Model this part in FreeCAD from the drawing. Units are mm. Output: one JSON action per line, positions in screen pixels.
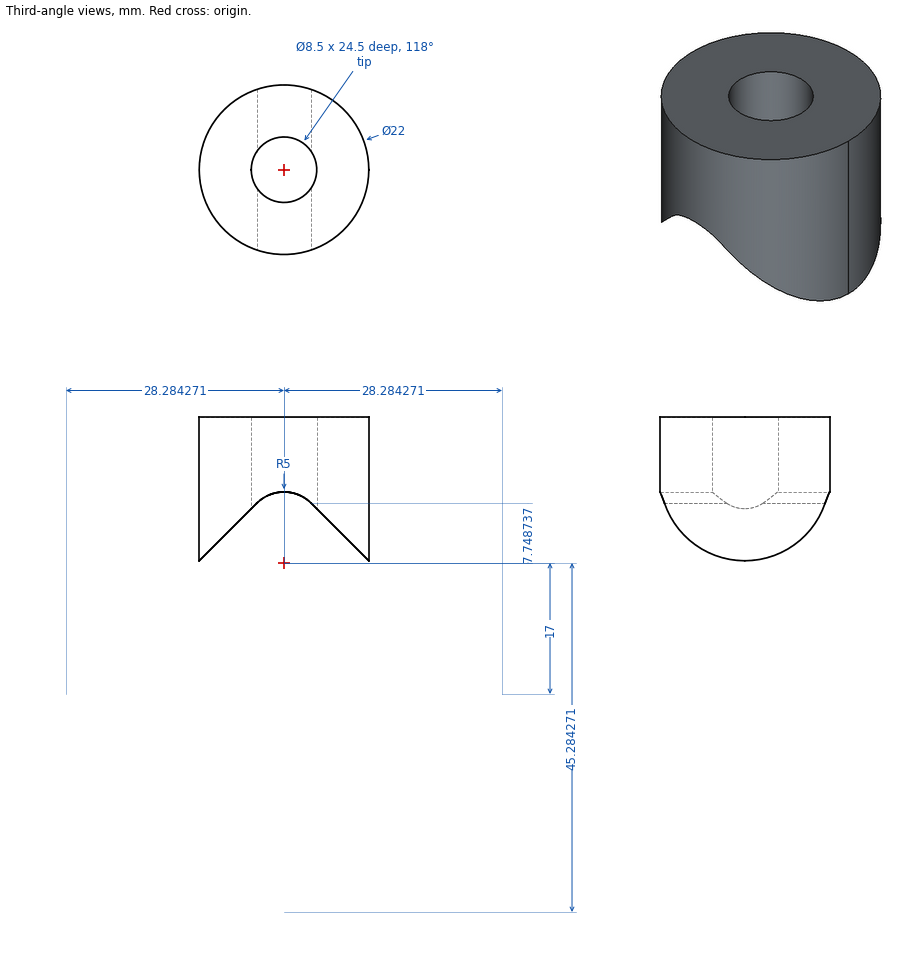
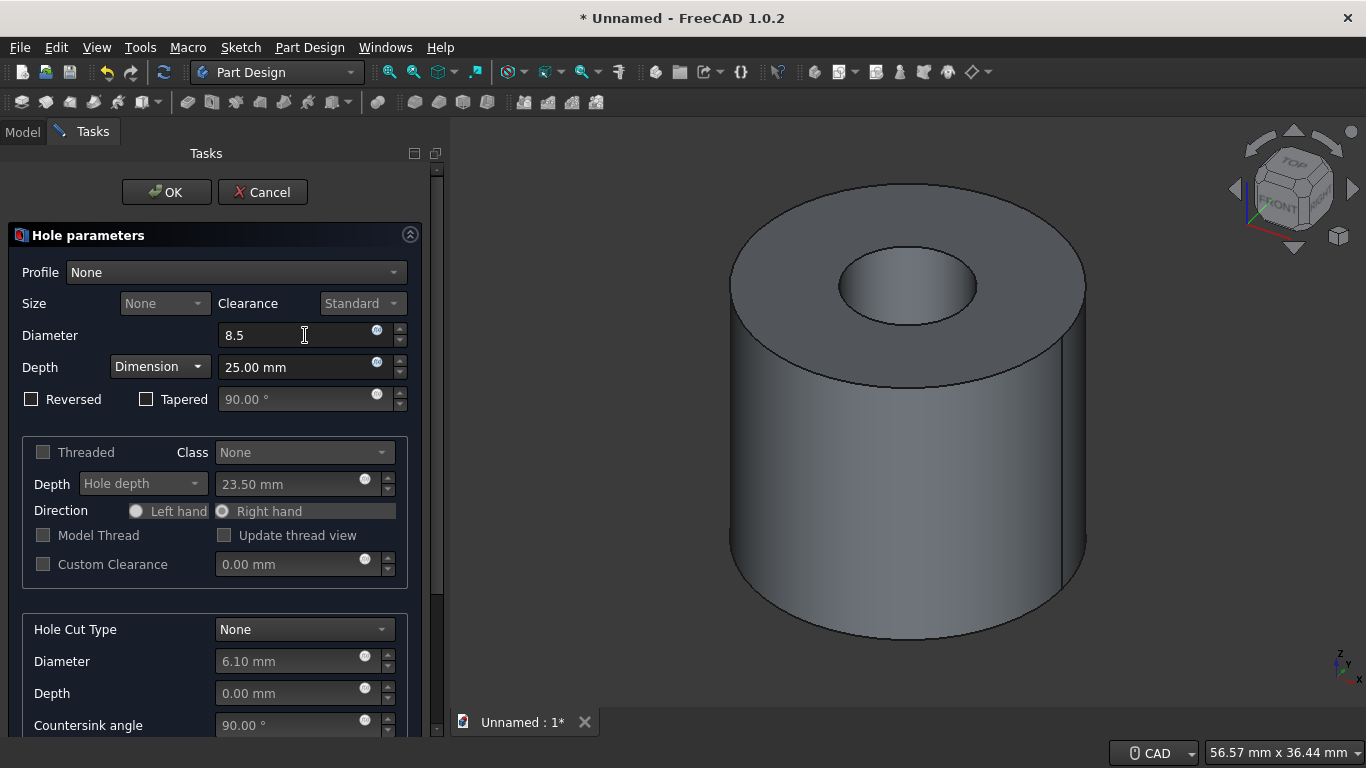
{"action": "triple_click", "coordinate": [305, 367]}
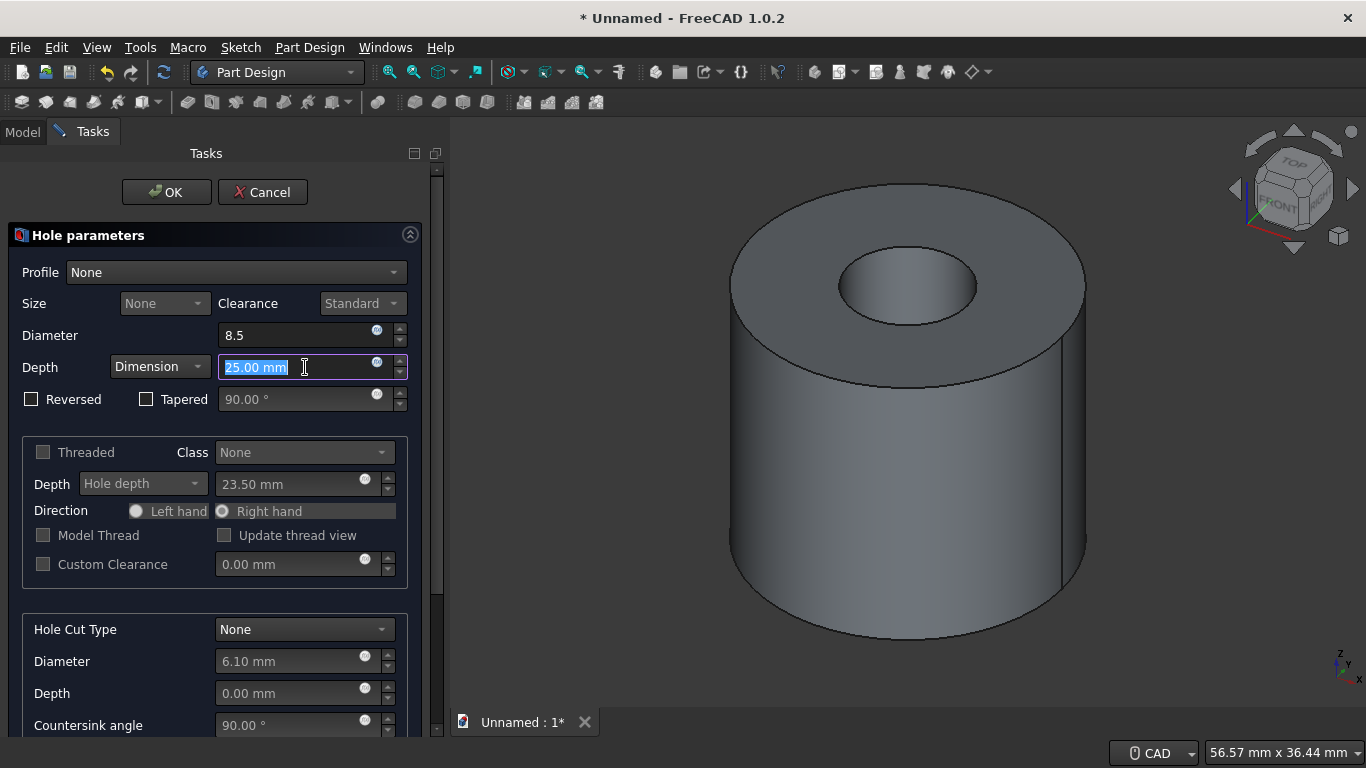
{"action": "type", "text": "24.5"}
{"action": "key", "text": "Tab"}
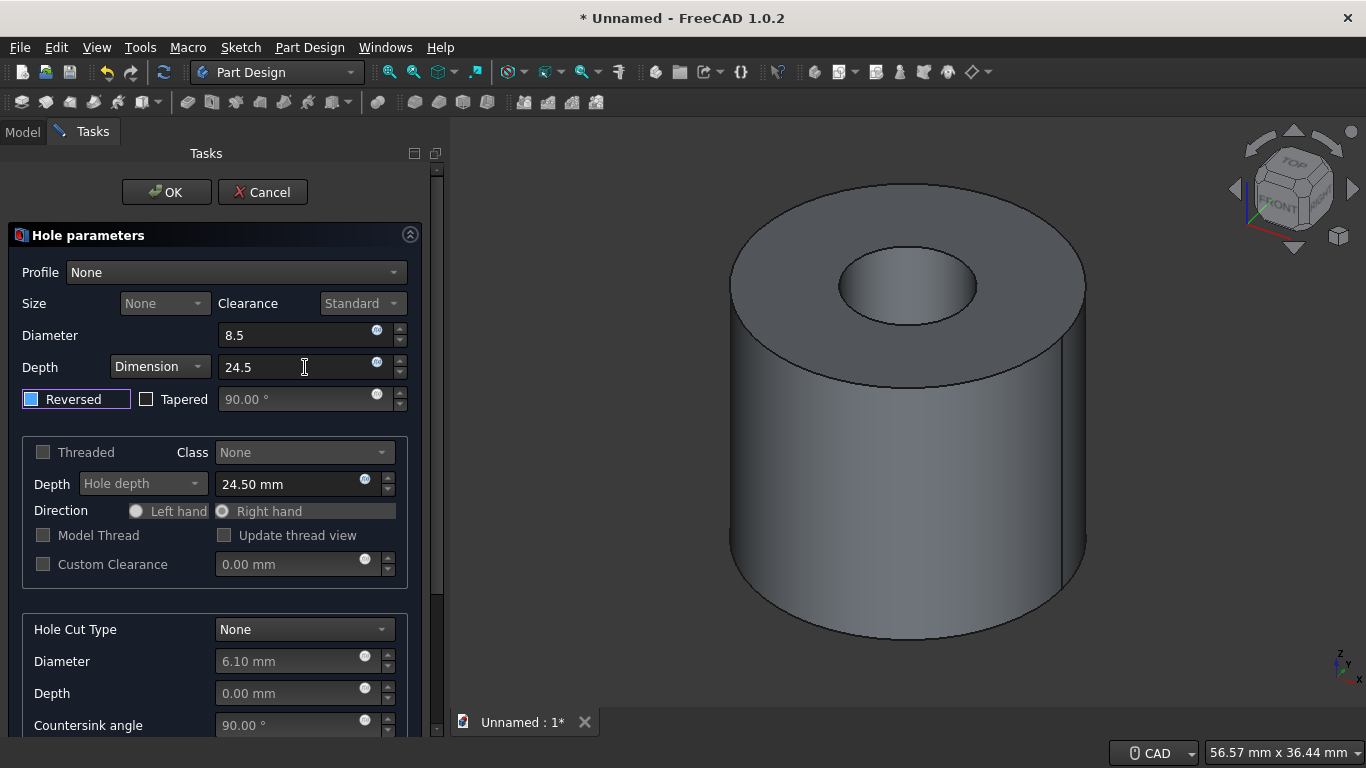
{"action": "left_click", "coordinate": [167, 192]}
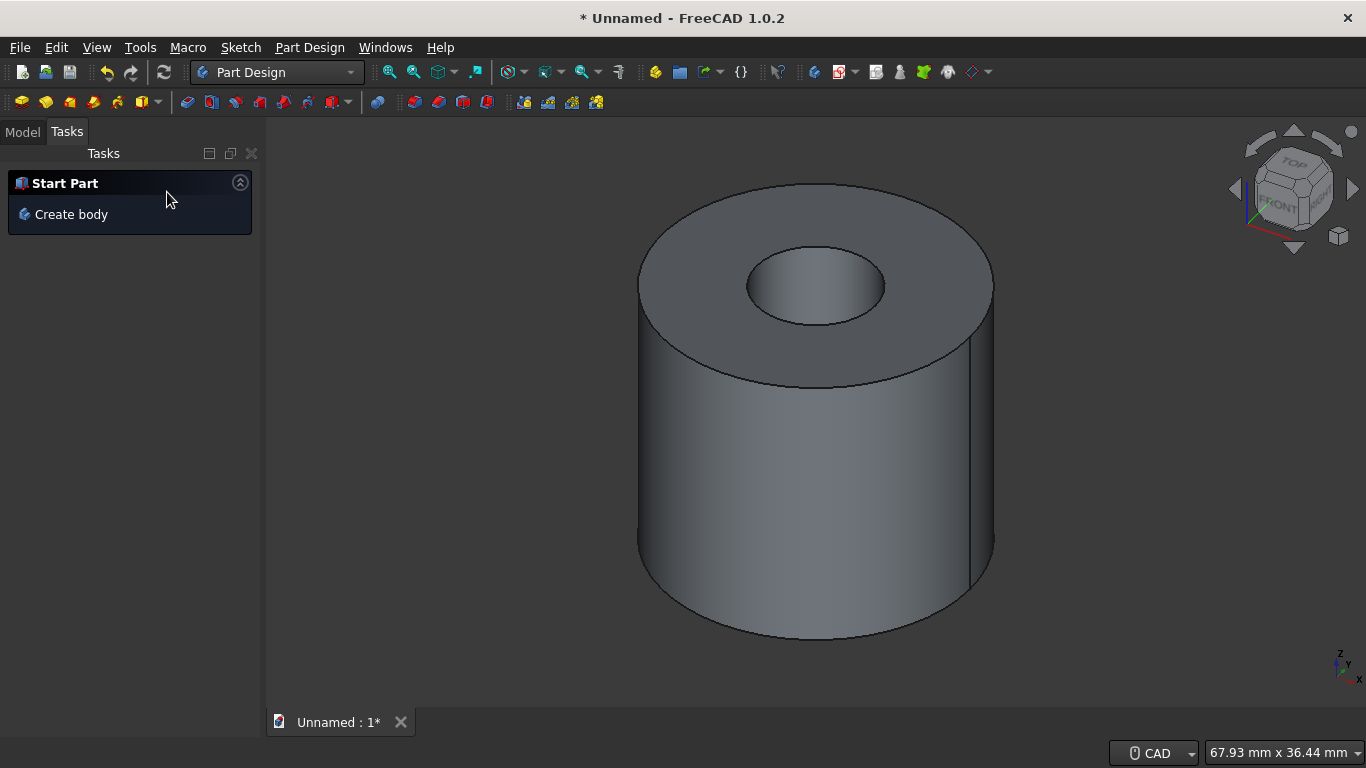
{"action": "left_click", "coordinate": [840, 72]}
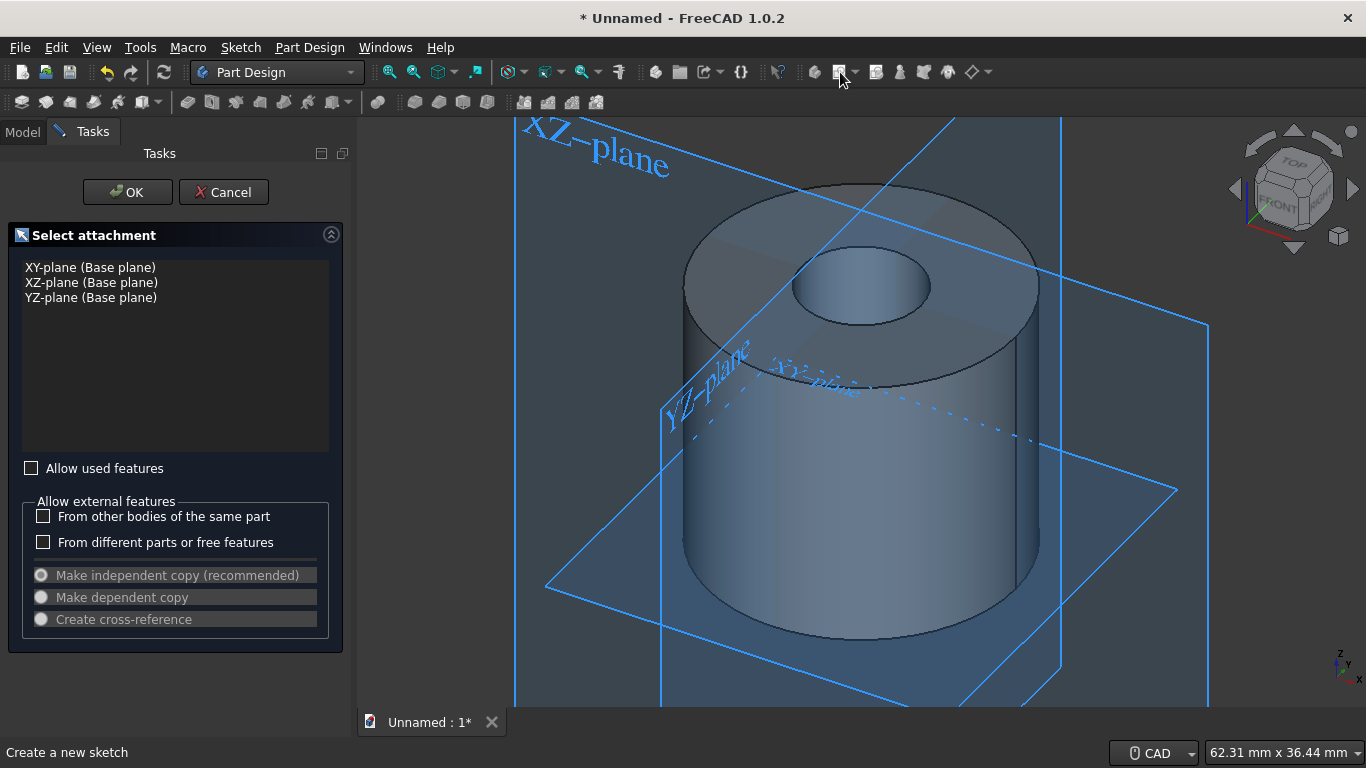
{"action": "left_click", "coordinate": [82, 282]}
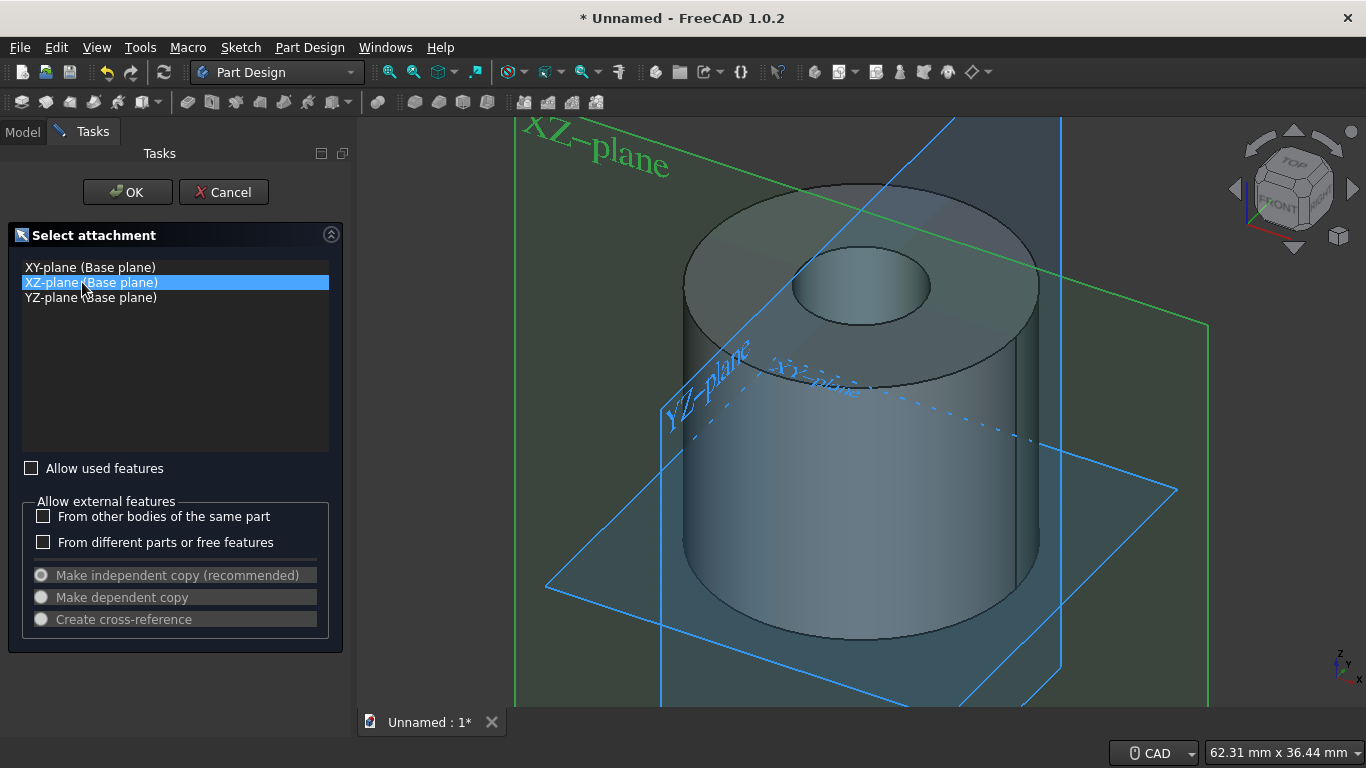
{"action": "left_click", "coordinate": [128, 192]}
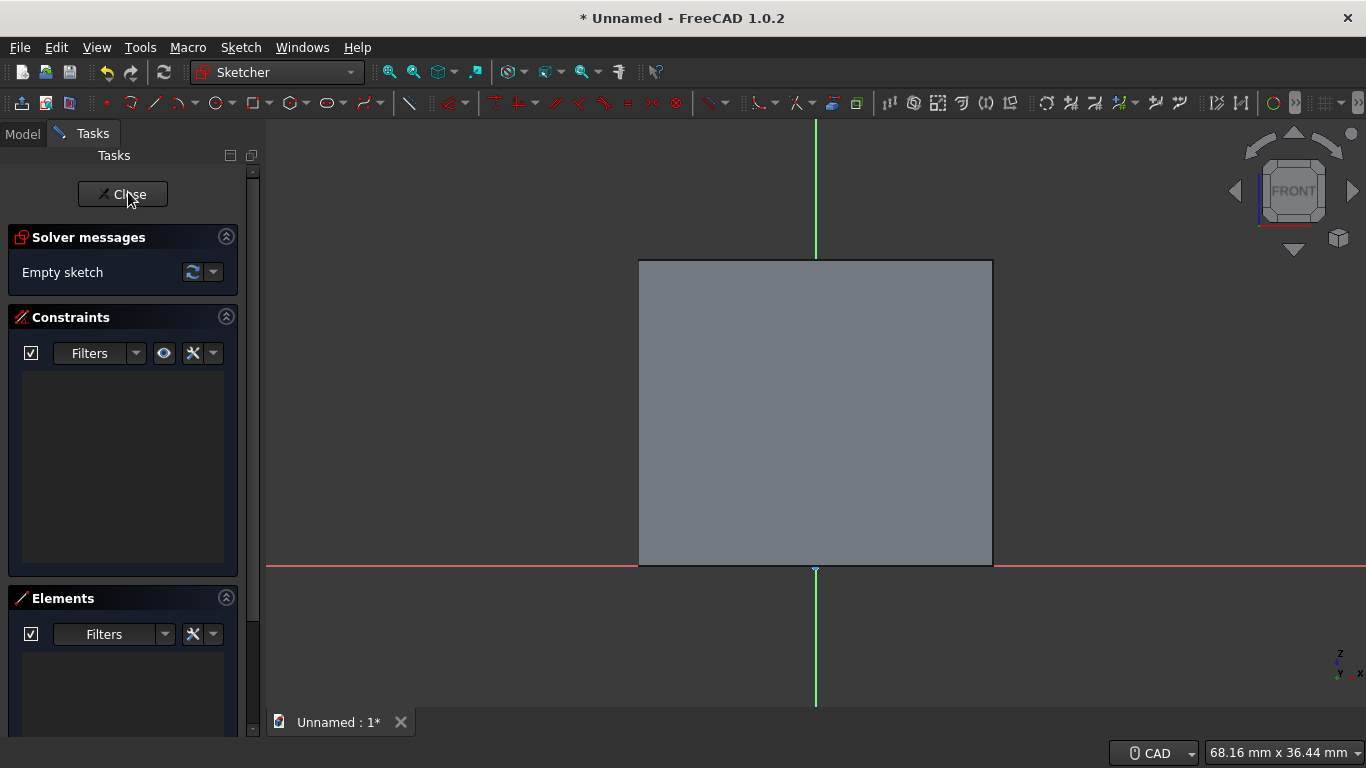
{"action": "key", "text": "q s"}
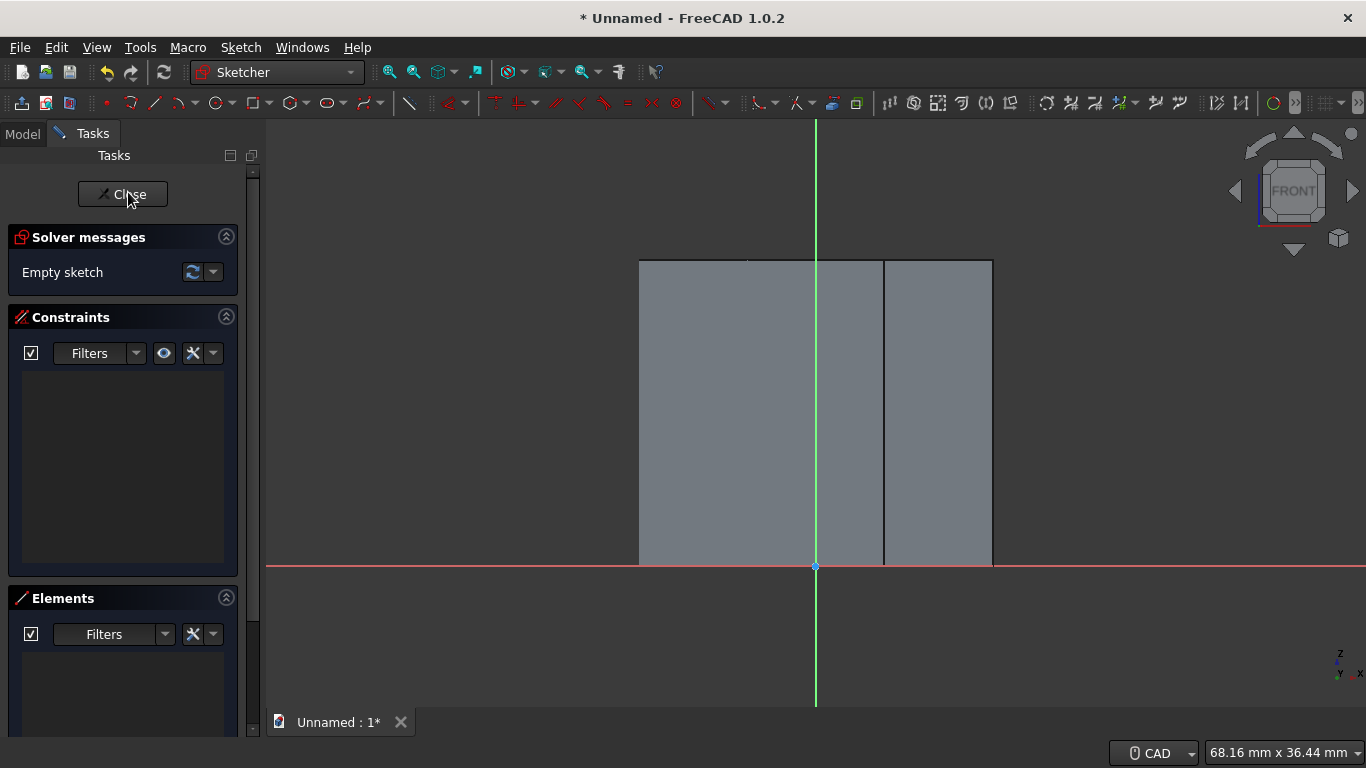
{"action": "scroll", "coordinate": [708, 154], "scroll_direction": "down", "scroll_amount": 5}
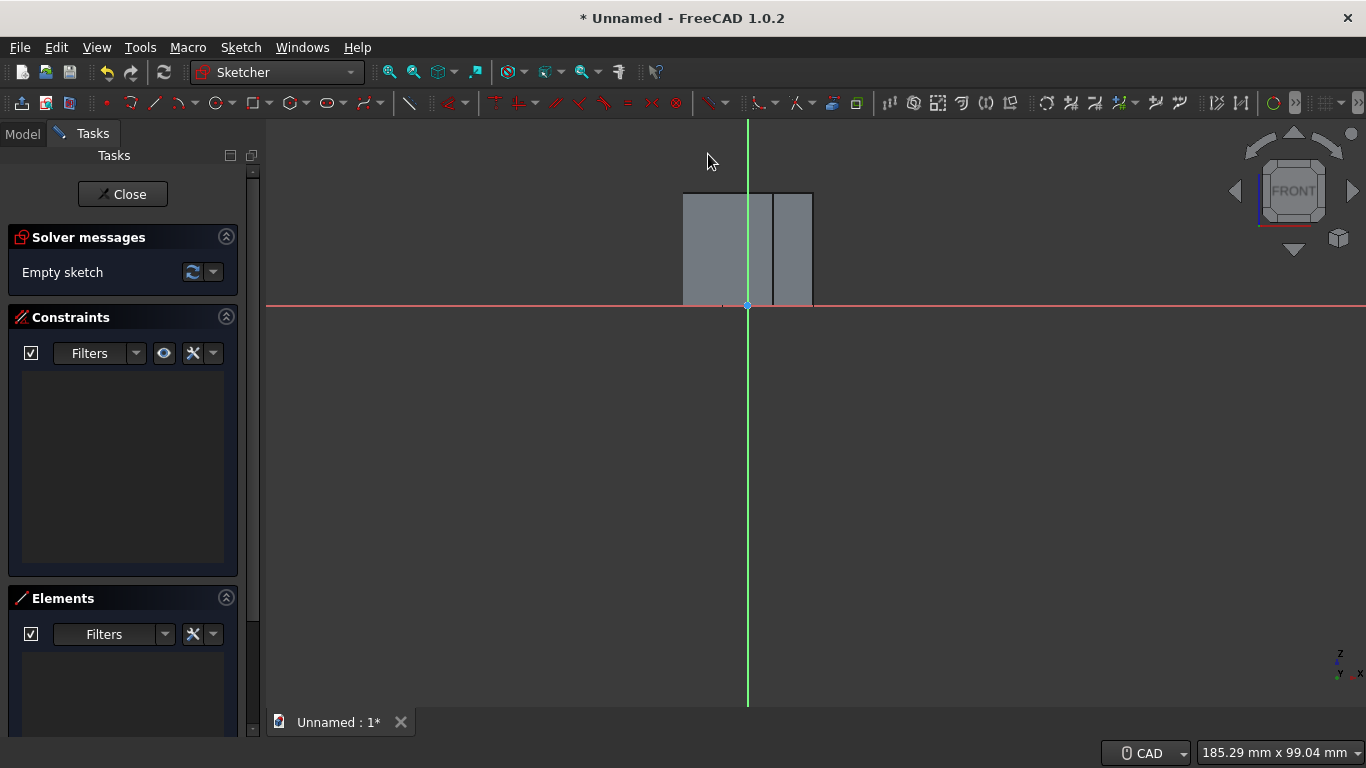
{"action": "key", "text": "g m"}